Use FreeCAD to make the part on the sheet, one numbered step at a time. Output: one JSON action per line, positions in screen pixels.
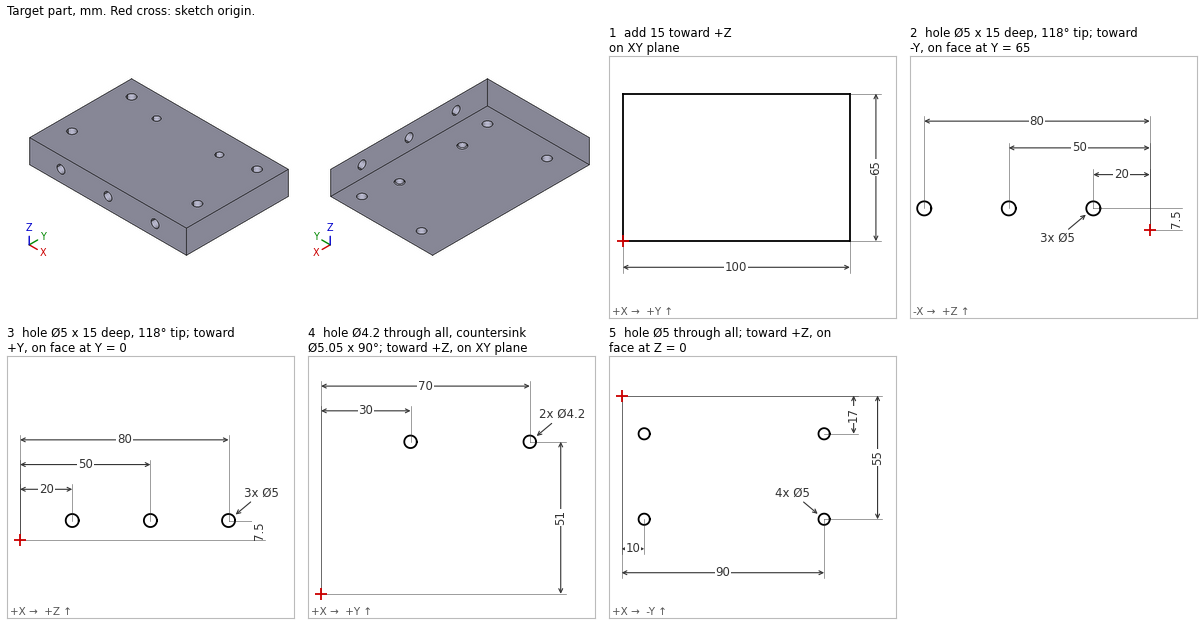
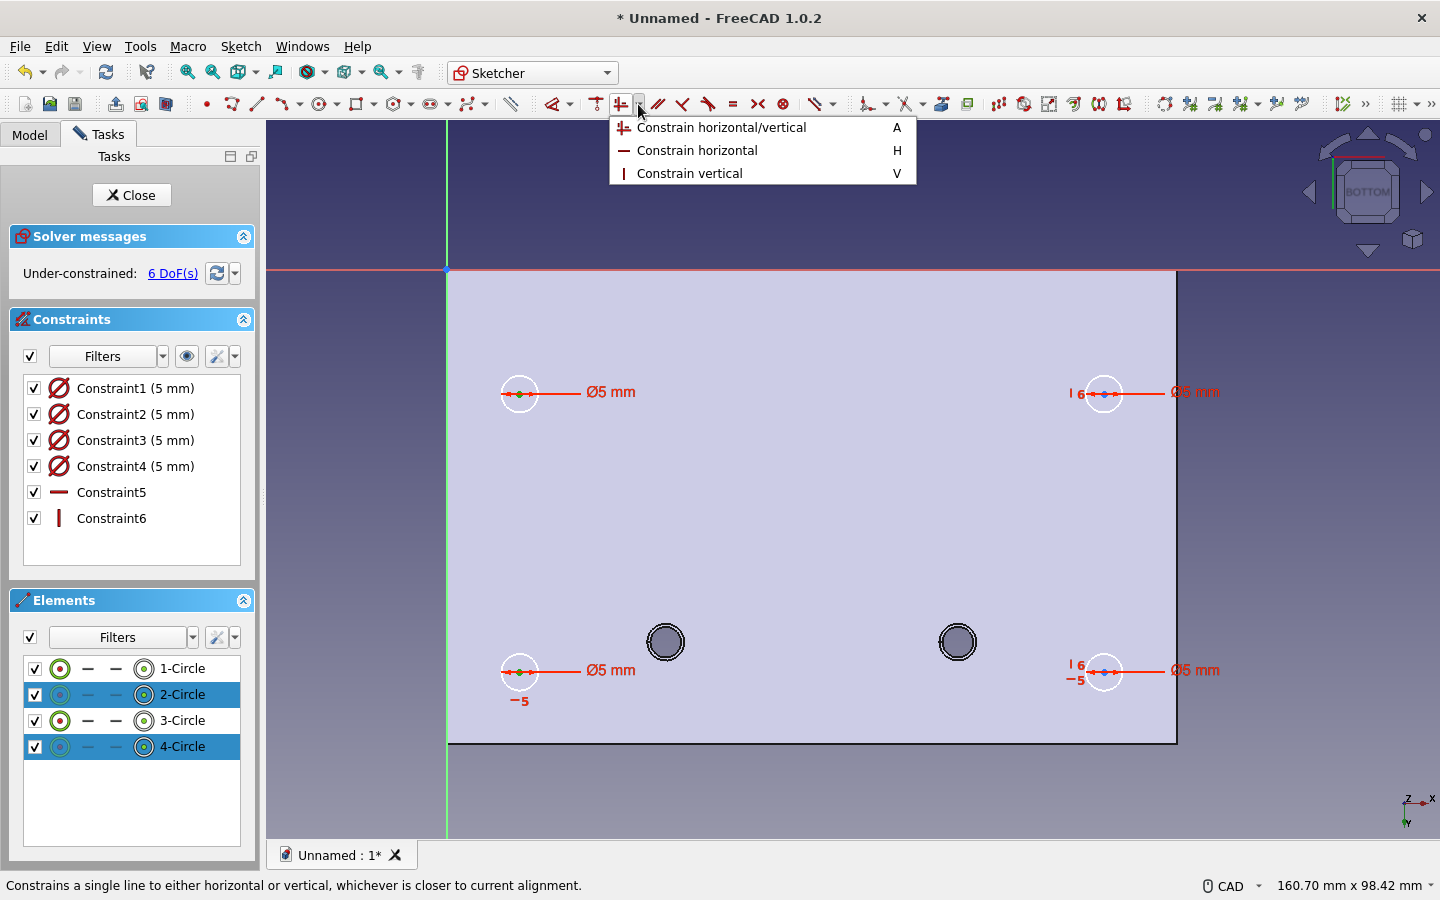
{"action": "left_click", "coordinate": [763, 174]}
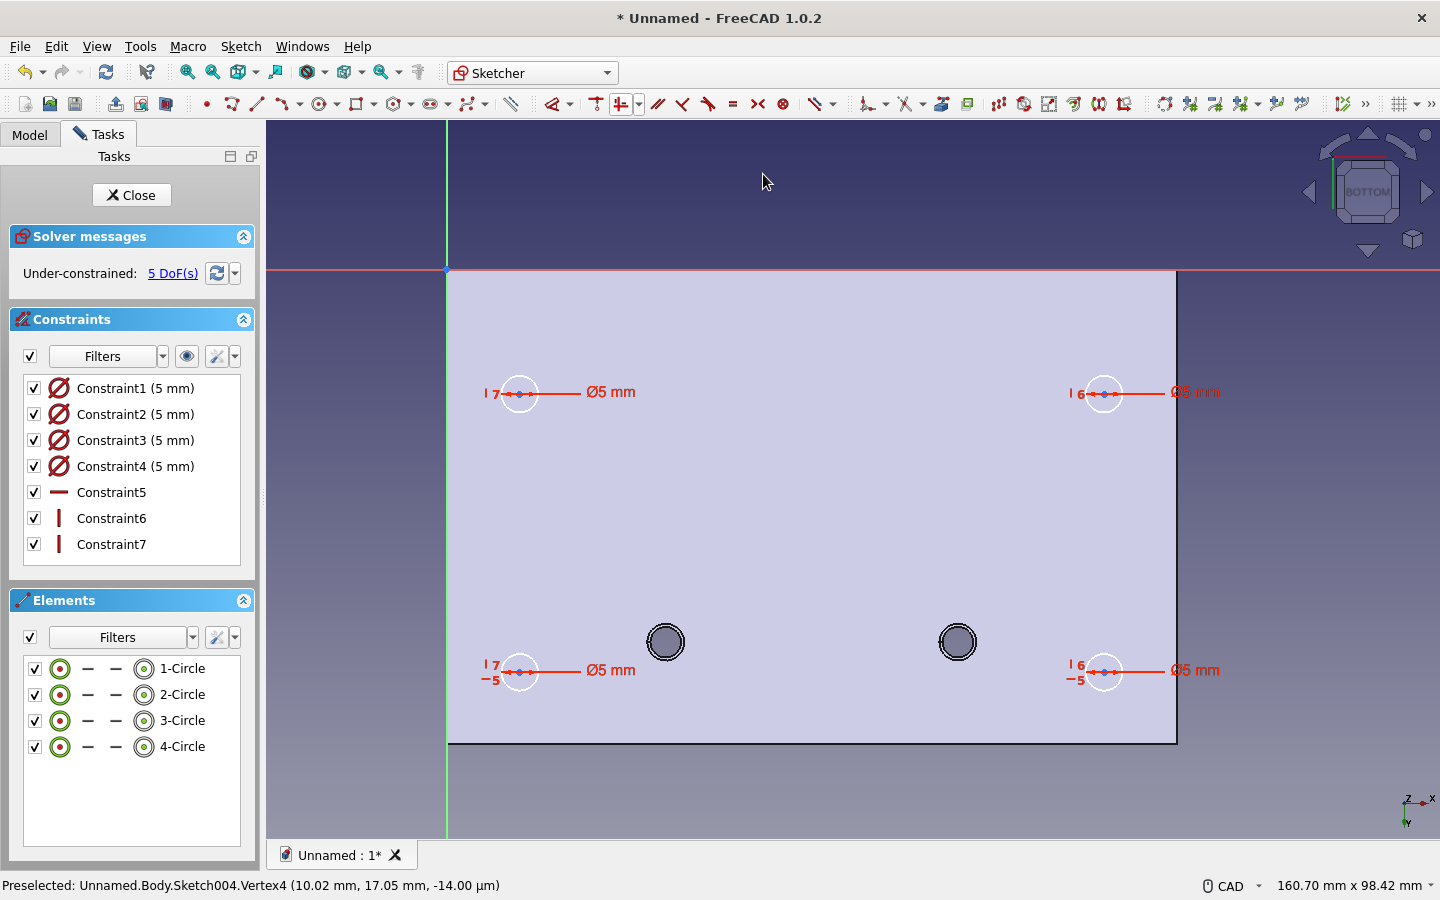
{"action": "left_click", "coordinate": [1104, 394]}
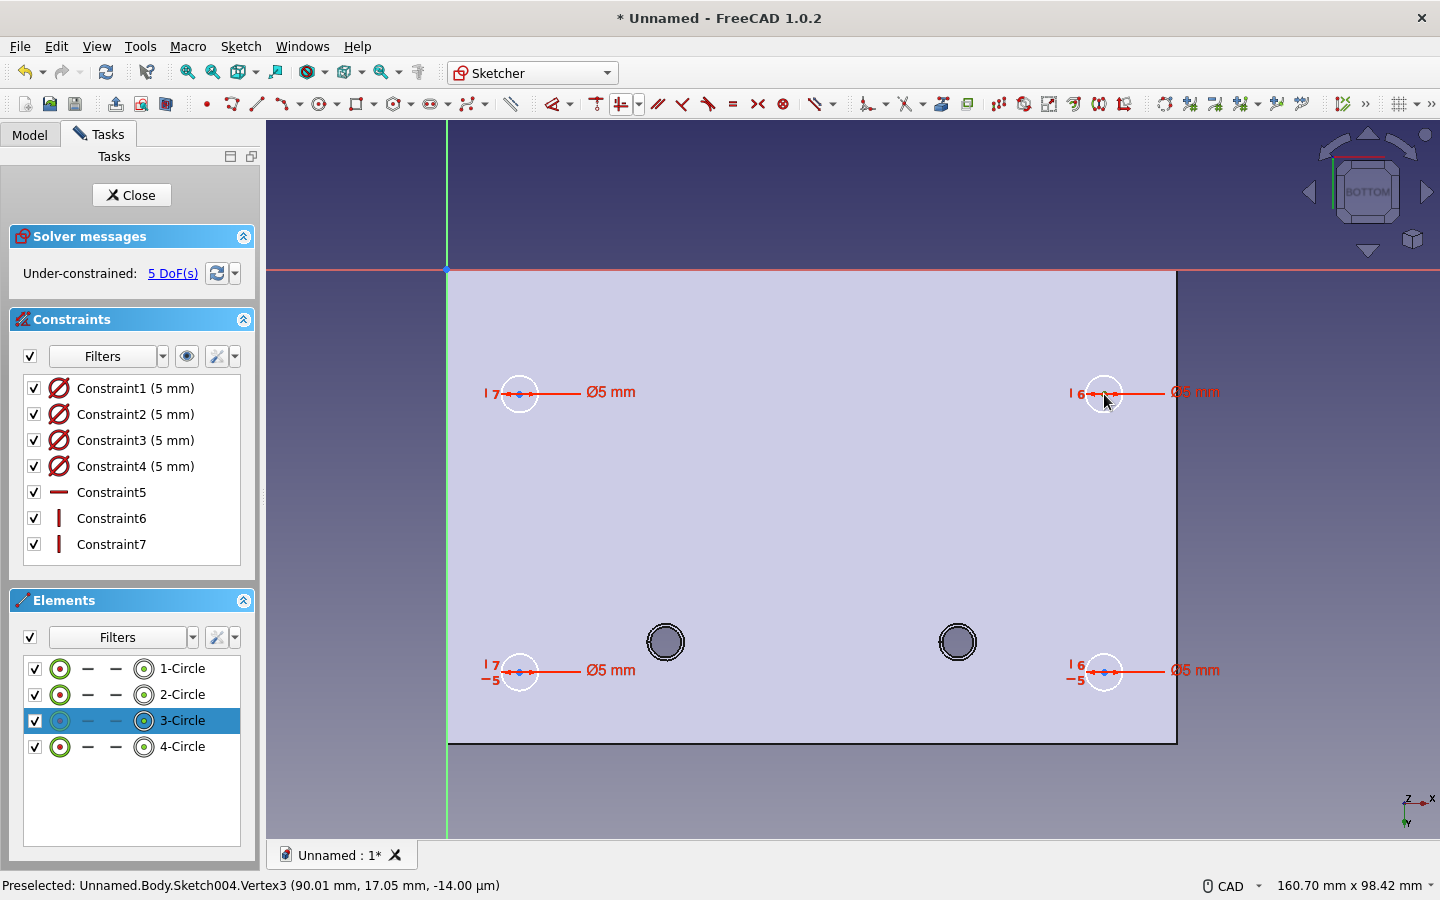
{"action": "left_click", "coordinate": [520, 394]}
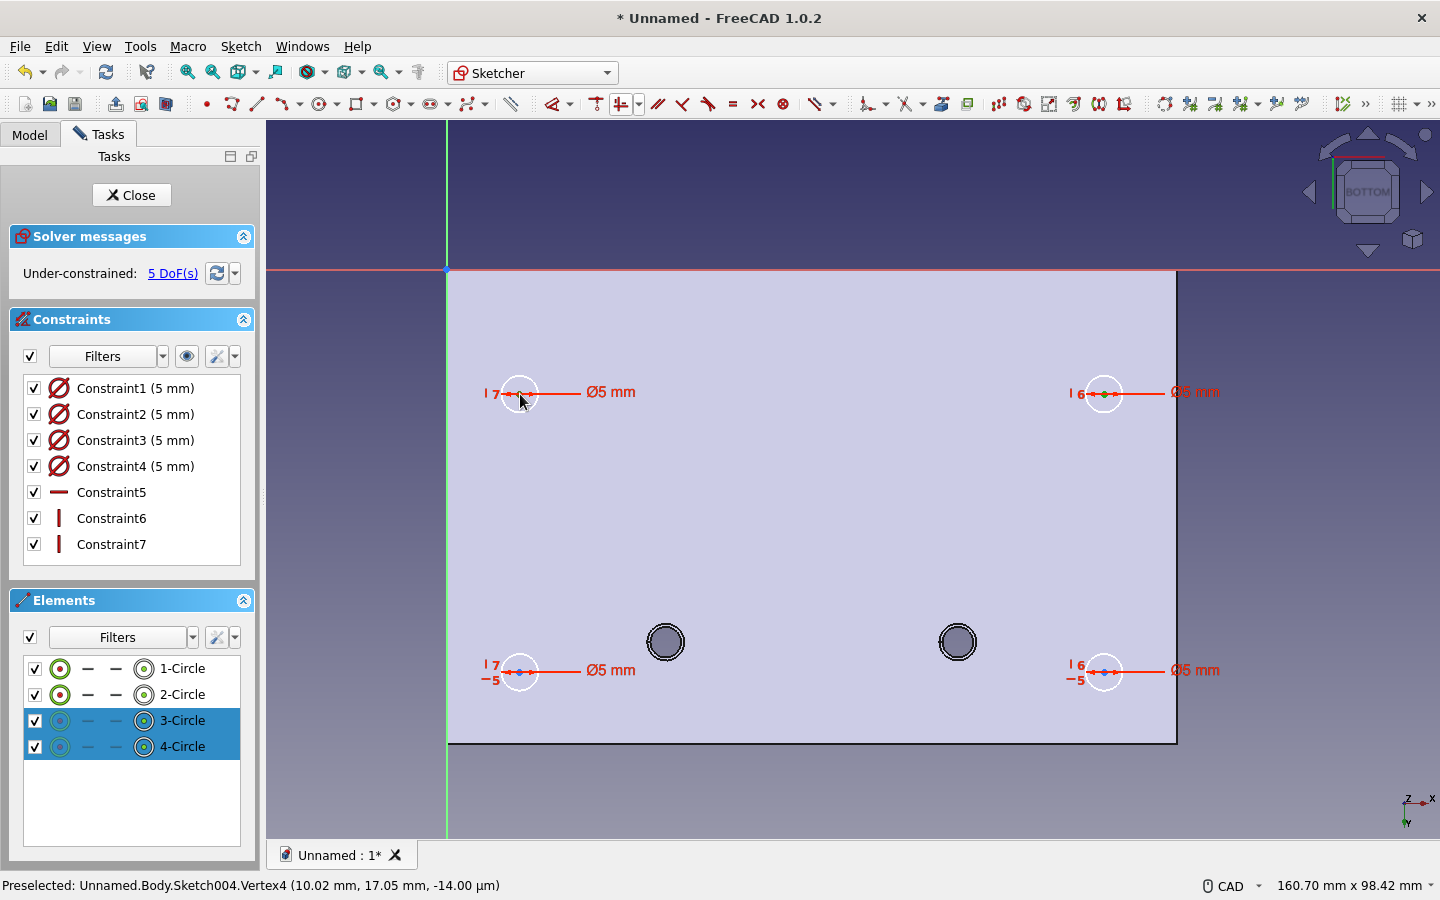
{"action": "key", "text": "h"}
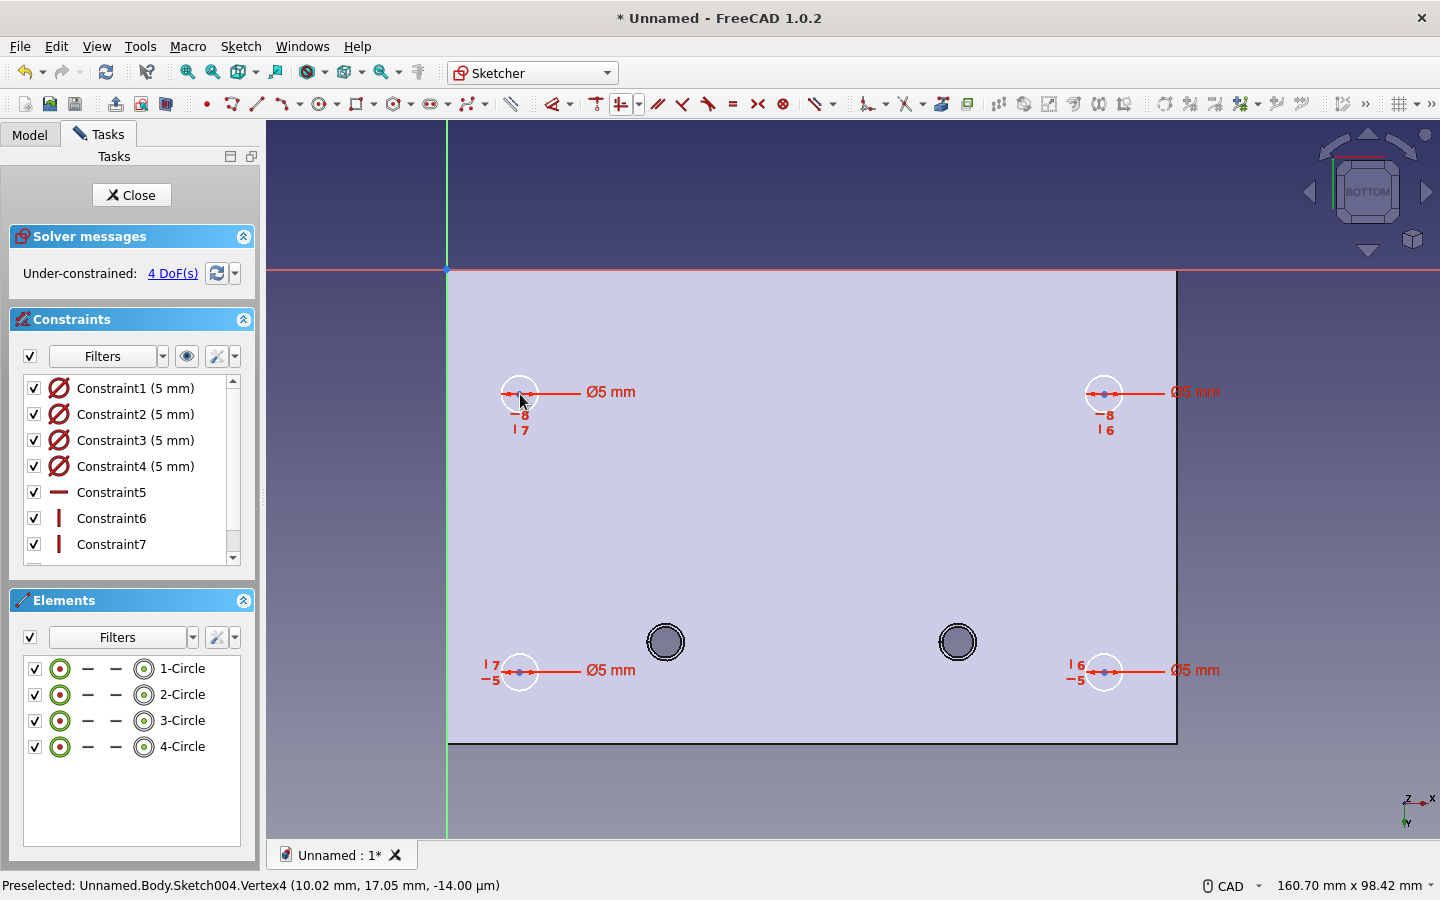
{"action": "key", "text": "d"}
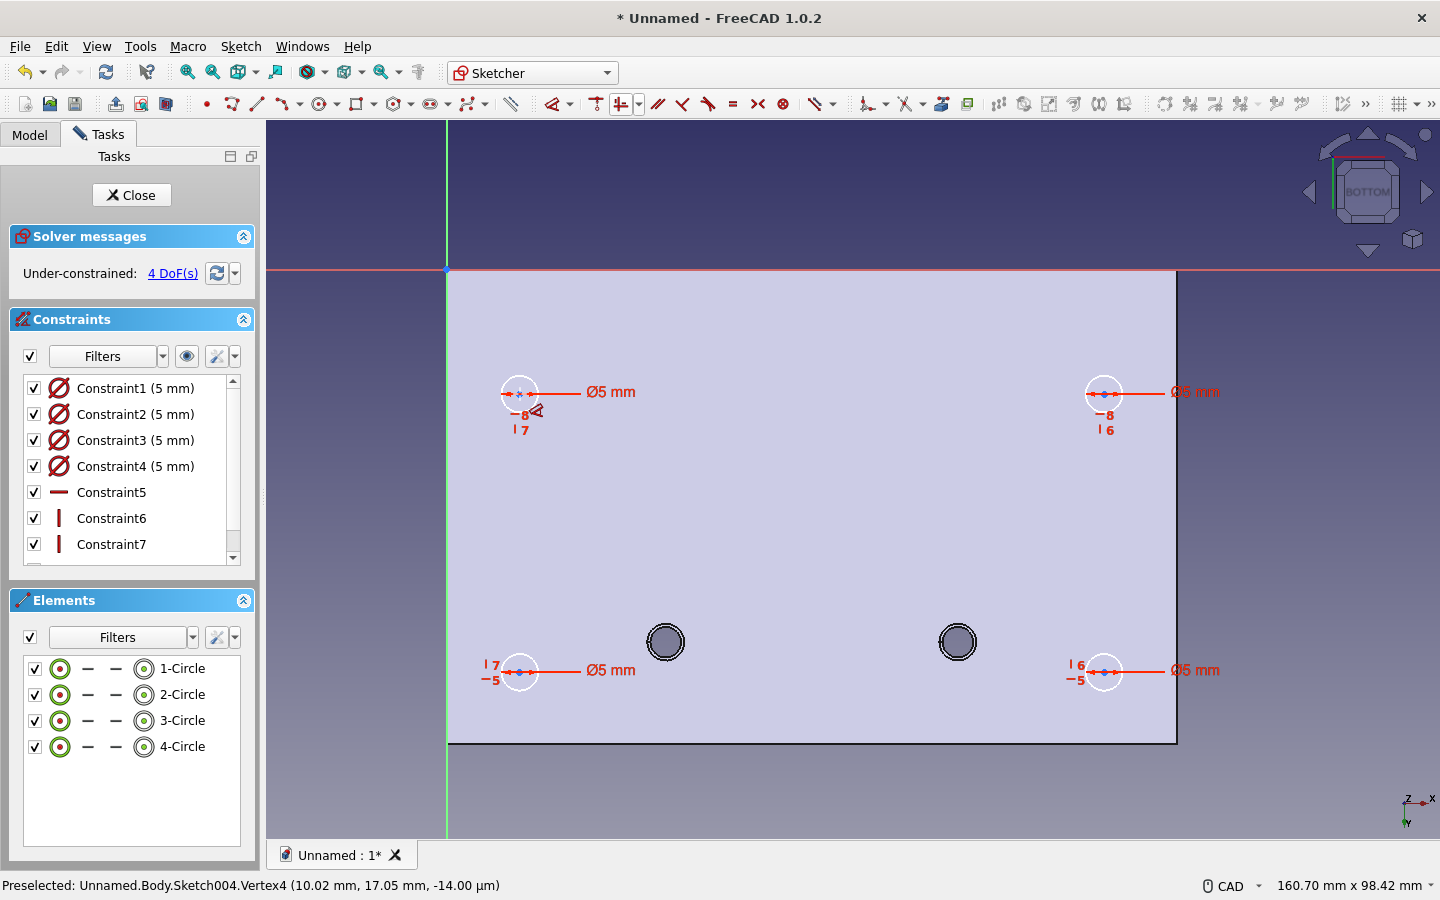
{"action": "left_click", "coordinate": [1104, 672]}
{"action": "left_click", "coordinate": [775, 236]}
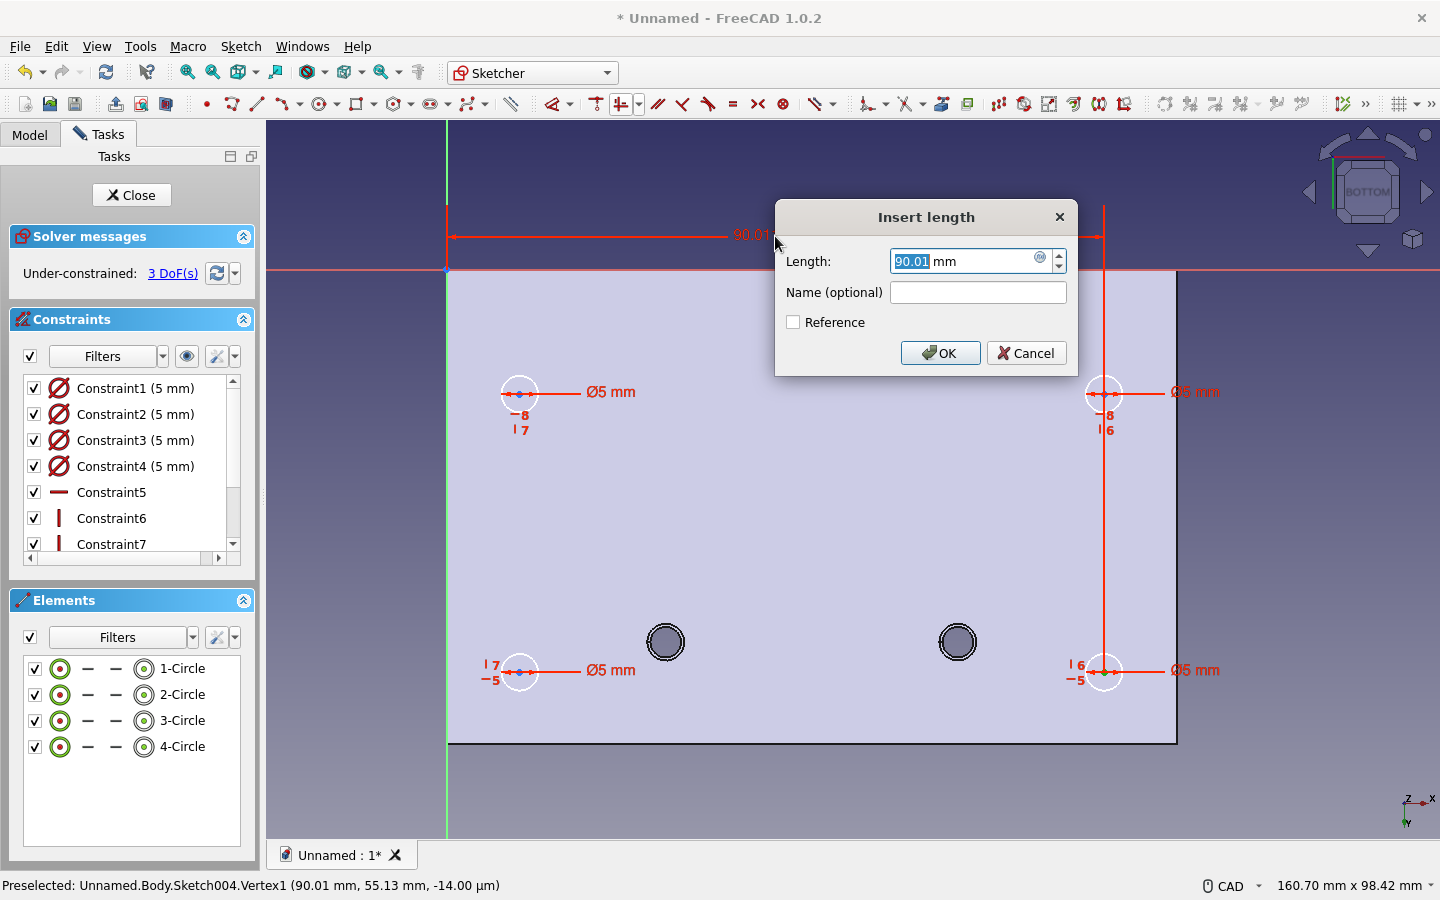
{"action": "type", "text": "90"}
{"action": "key", "text": "Return"}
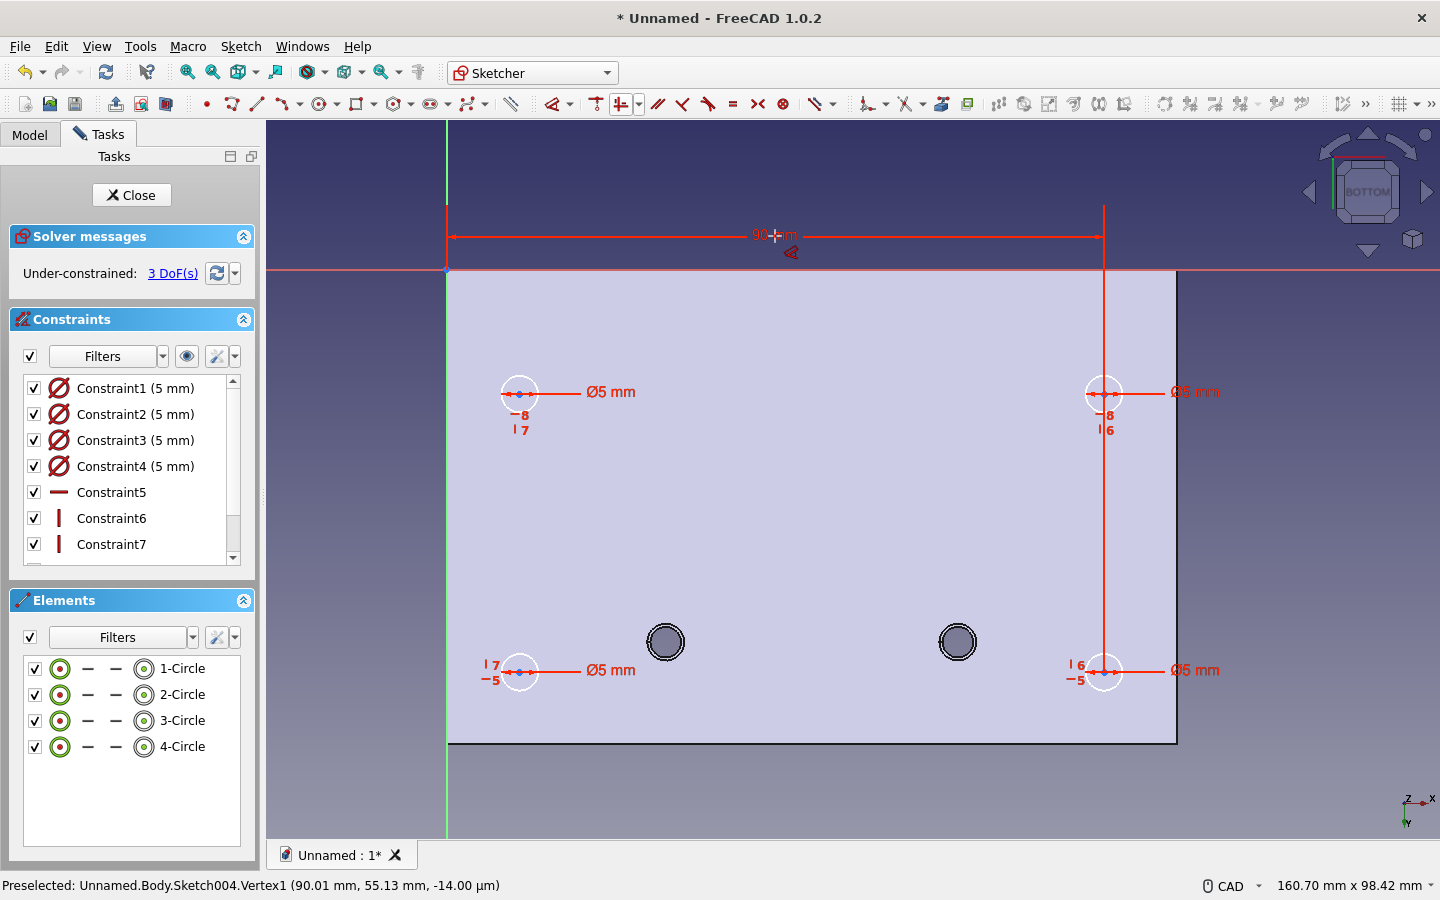
{"action": "left_click", "coordinate": [1104, 672]}
{"action": "left_click", "coordinate": [413, 471]}